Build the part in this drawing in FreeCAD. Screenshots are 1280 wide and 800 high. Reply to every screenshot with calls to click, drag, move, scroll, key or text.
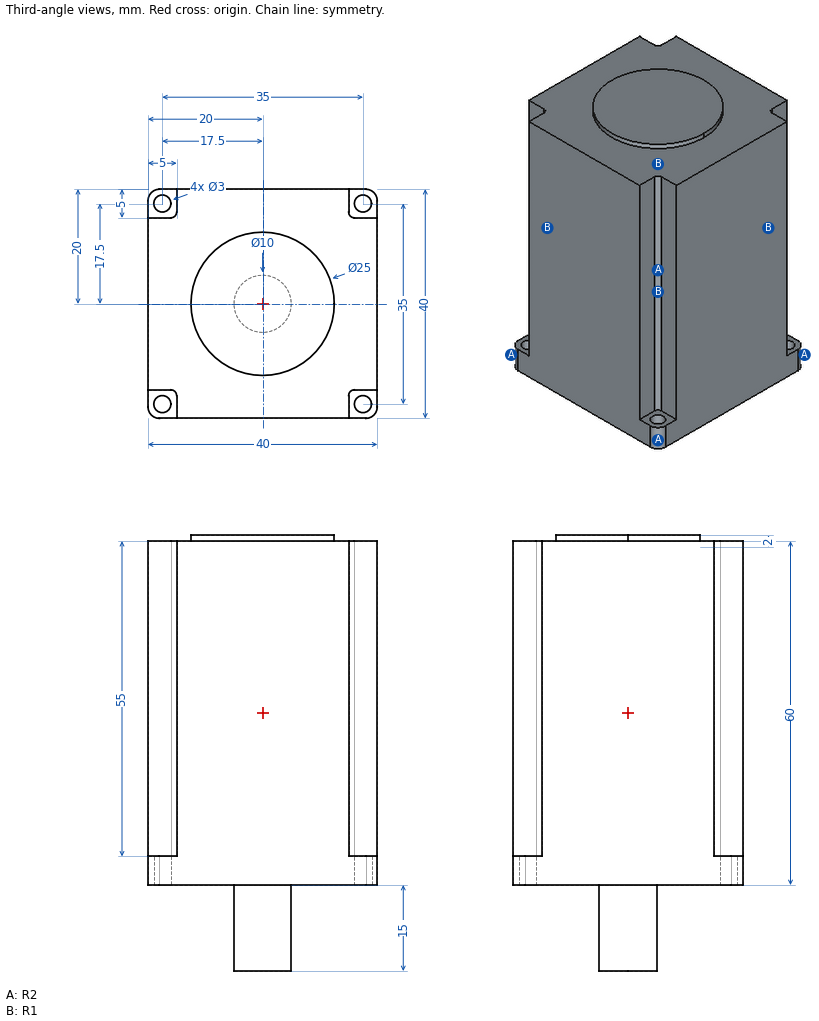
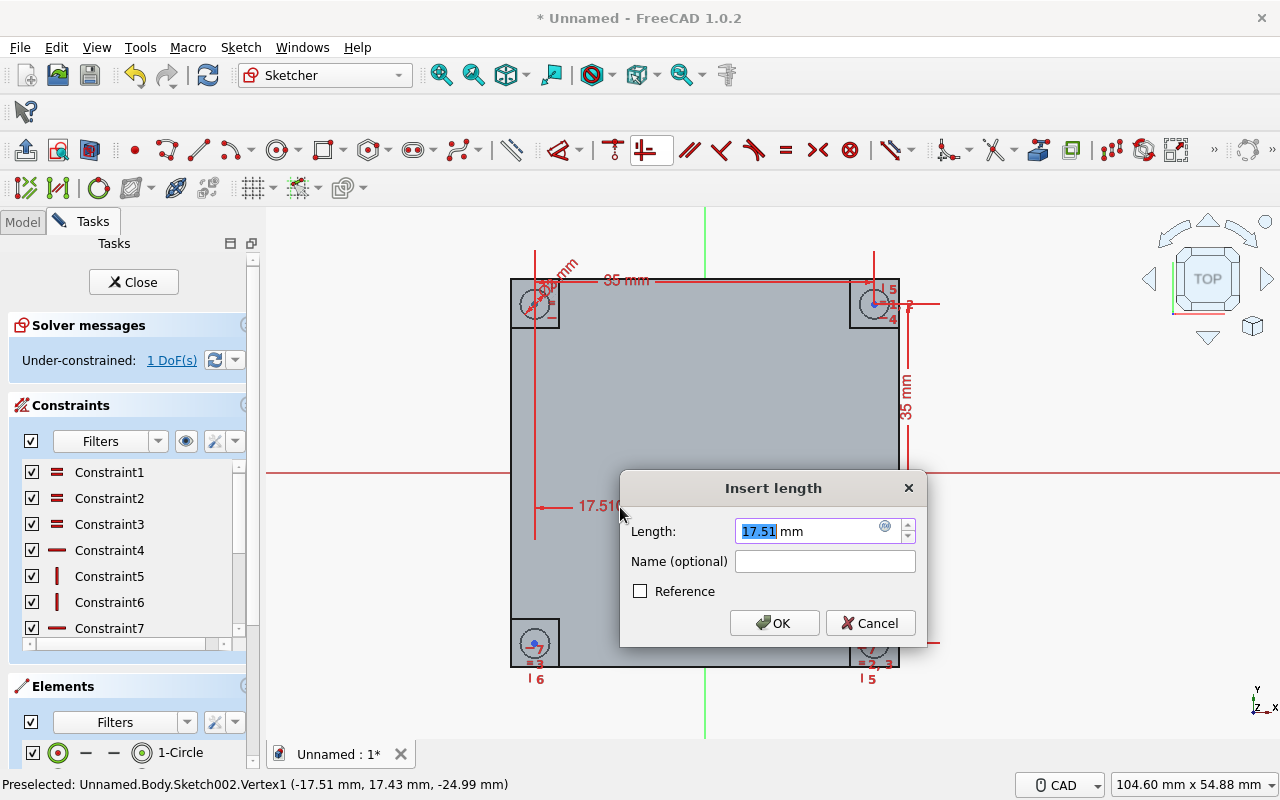
text(17.5)
key(Return)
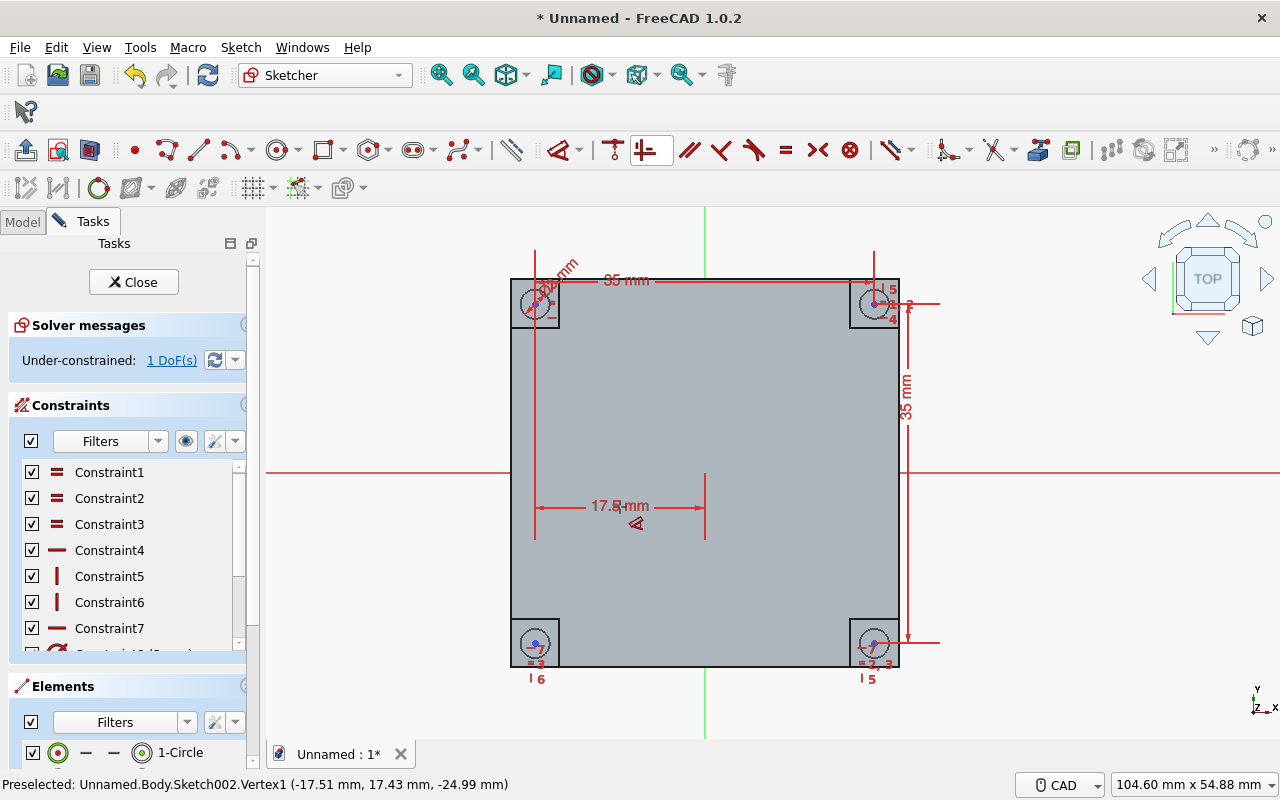
click(535, 304)
click(501, 389)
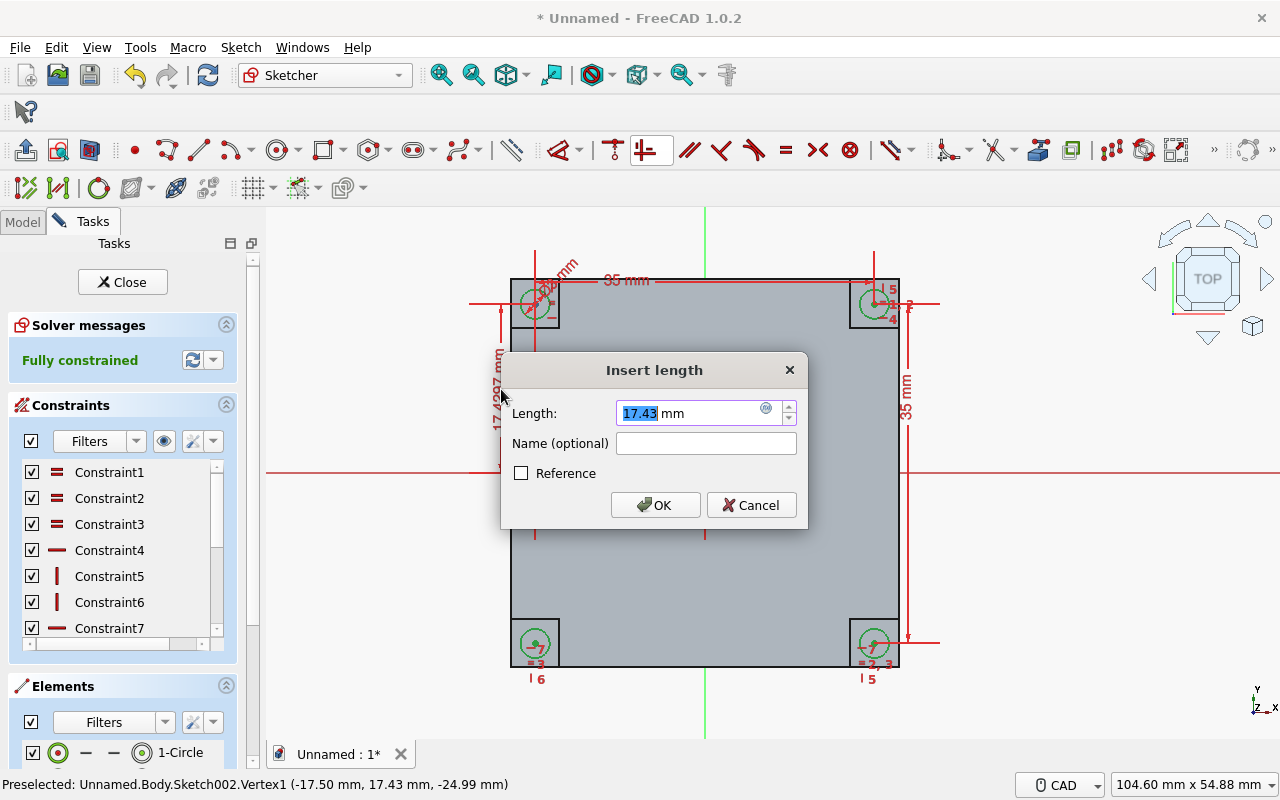
text(17.5)
key(Return)
key(Escape)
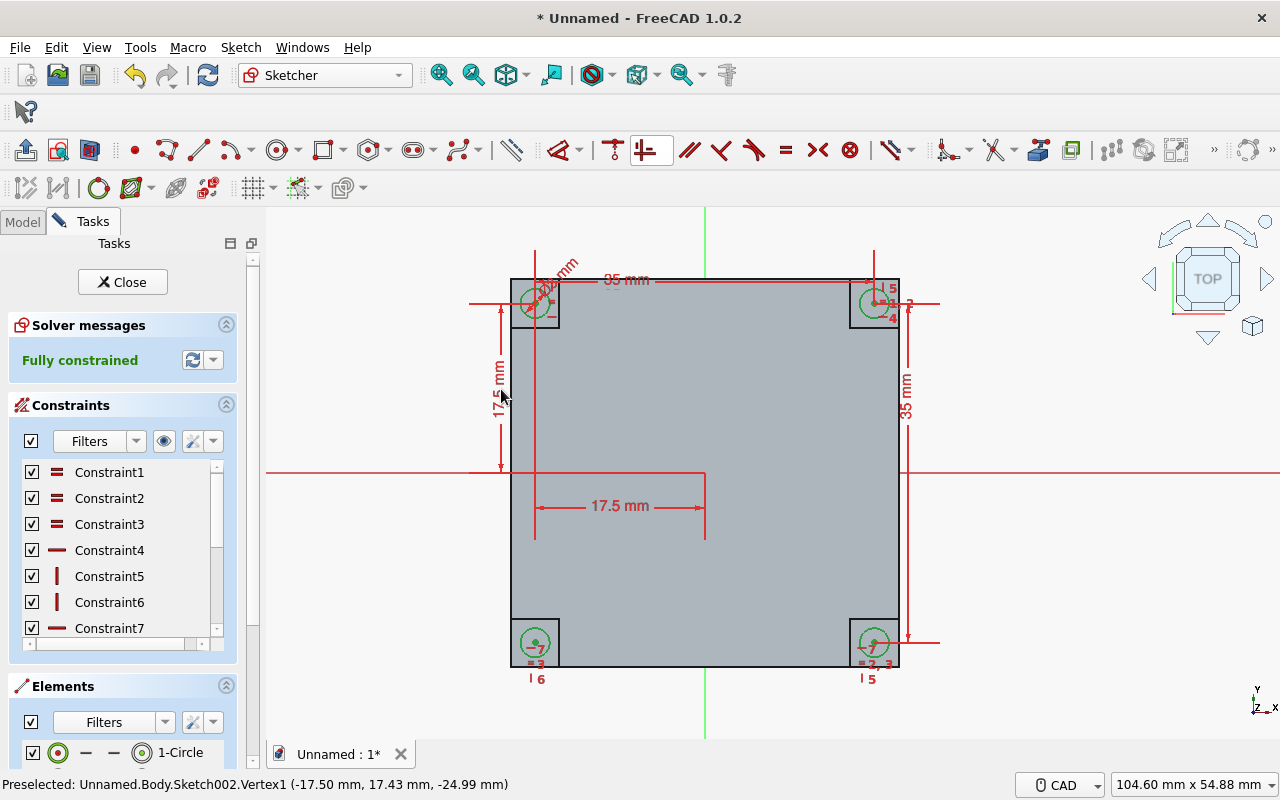
click(123, 282)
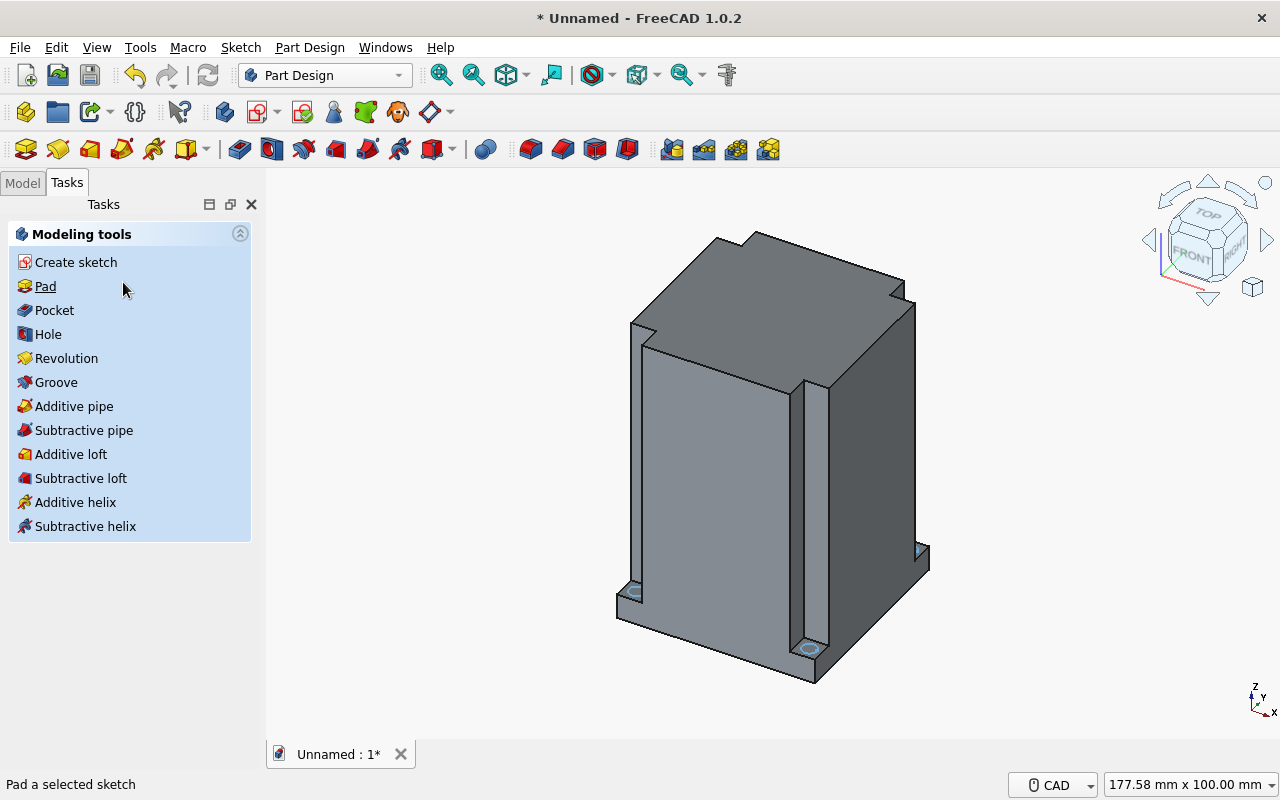
click(240, 150)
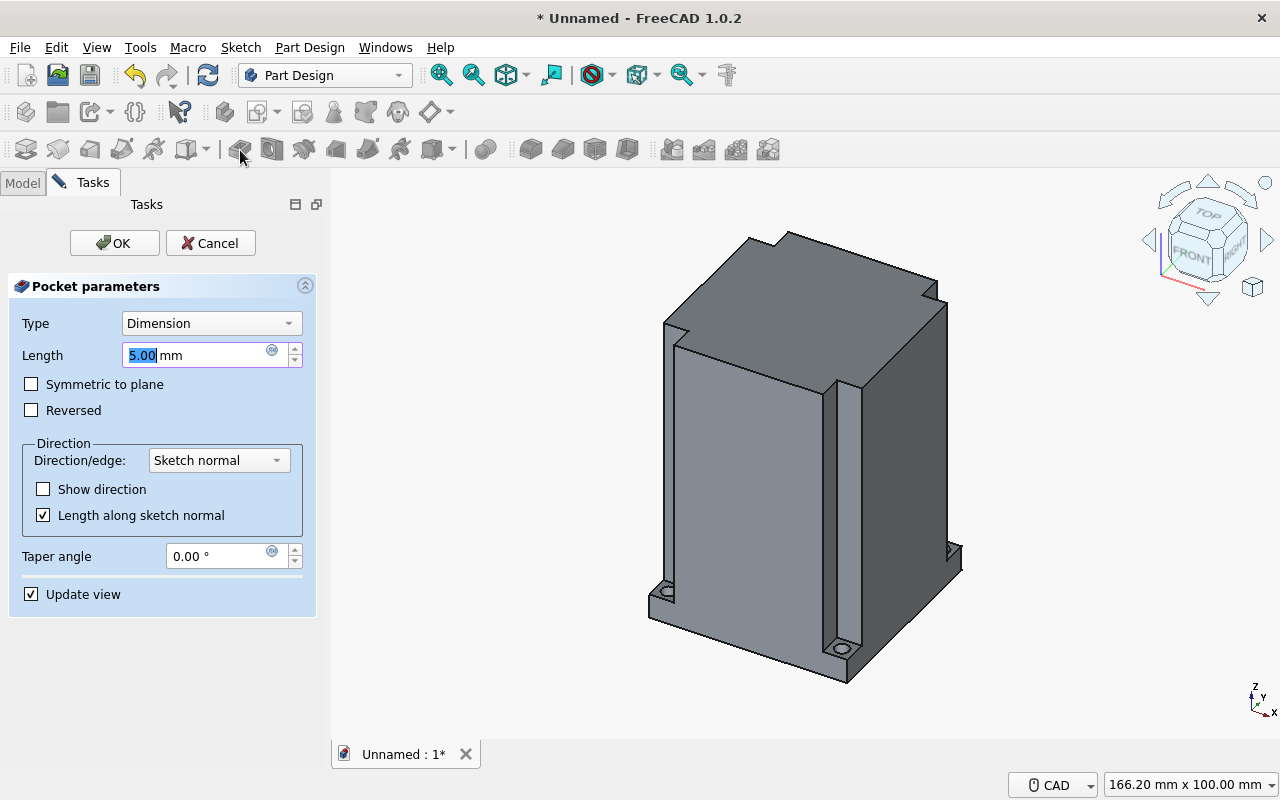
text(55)
key(Tab)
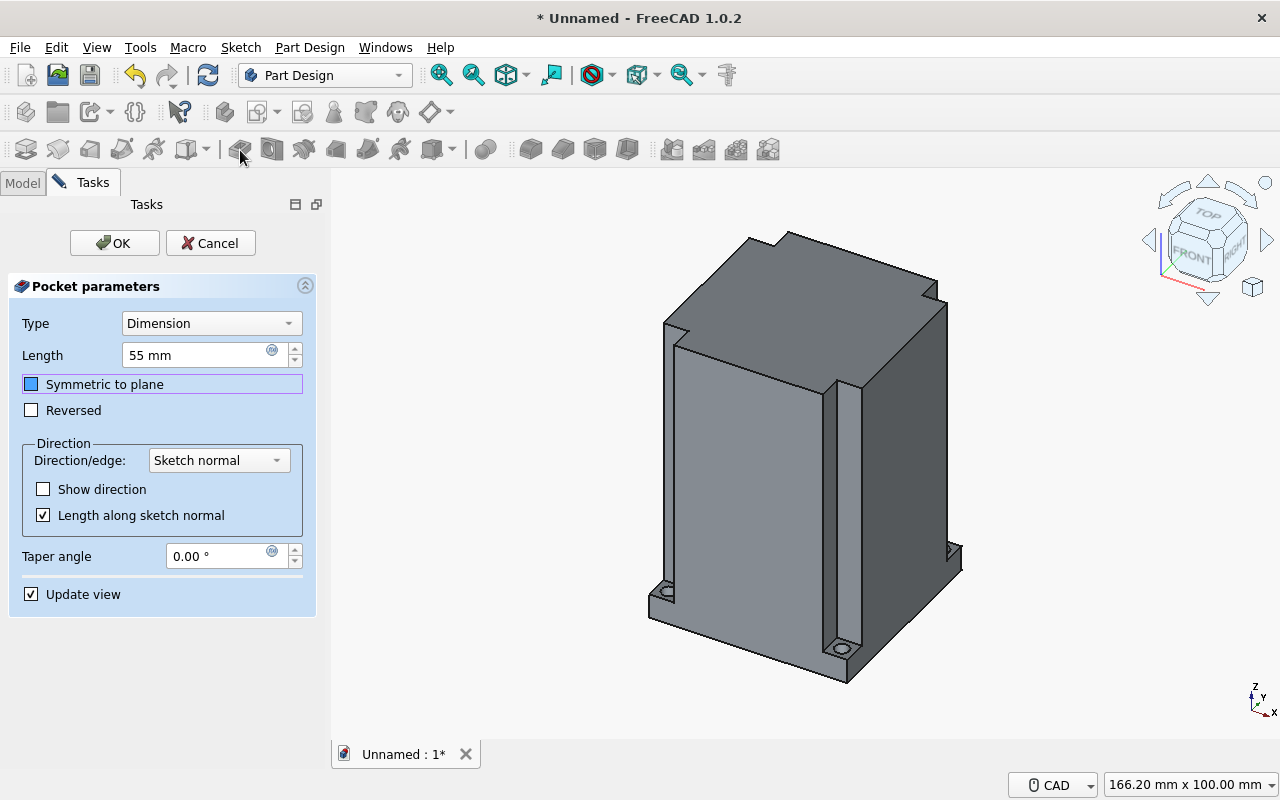
click(115, 243)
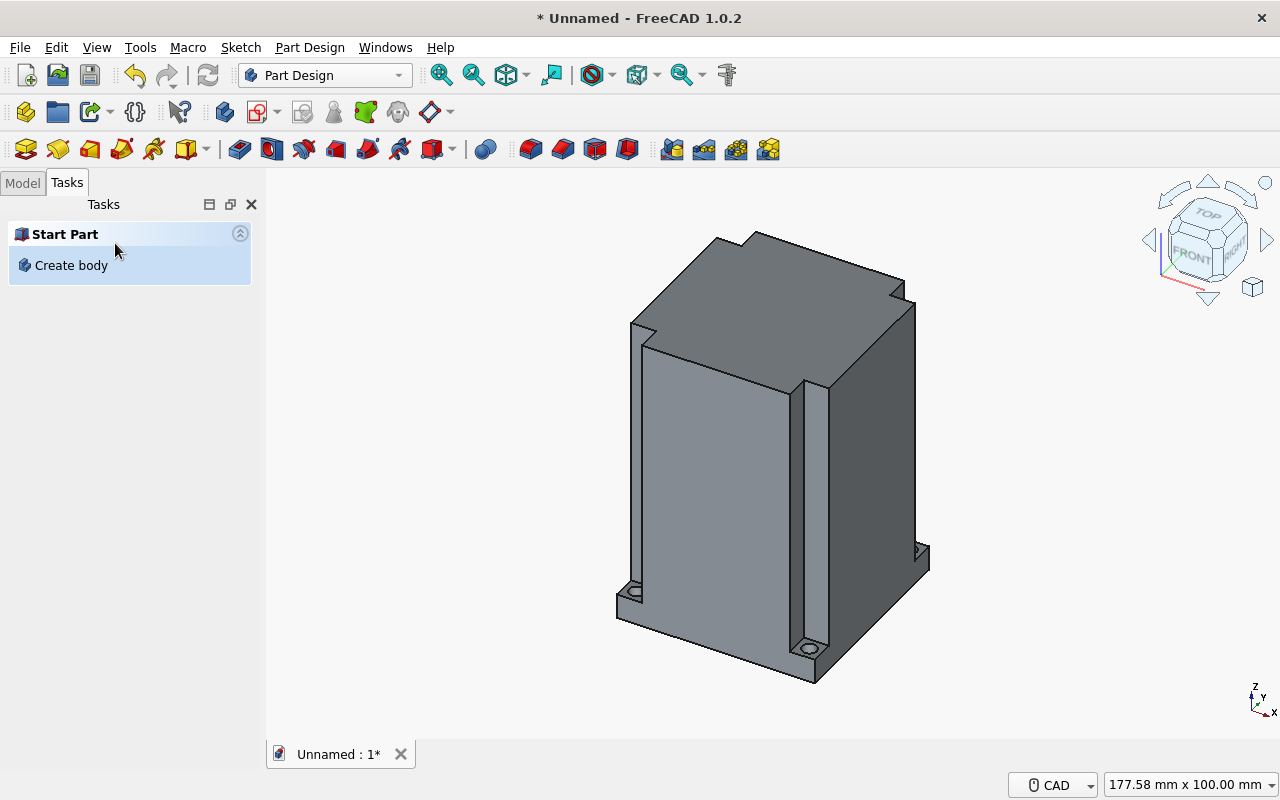
click(815, 671)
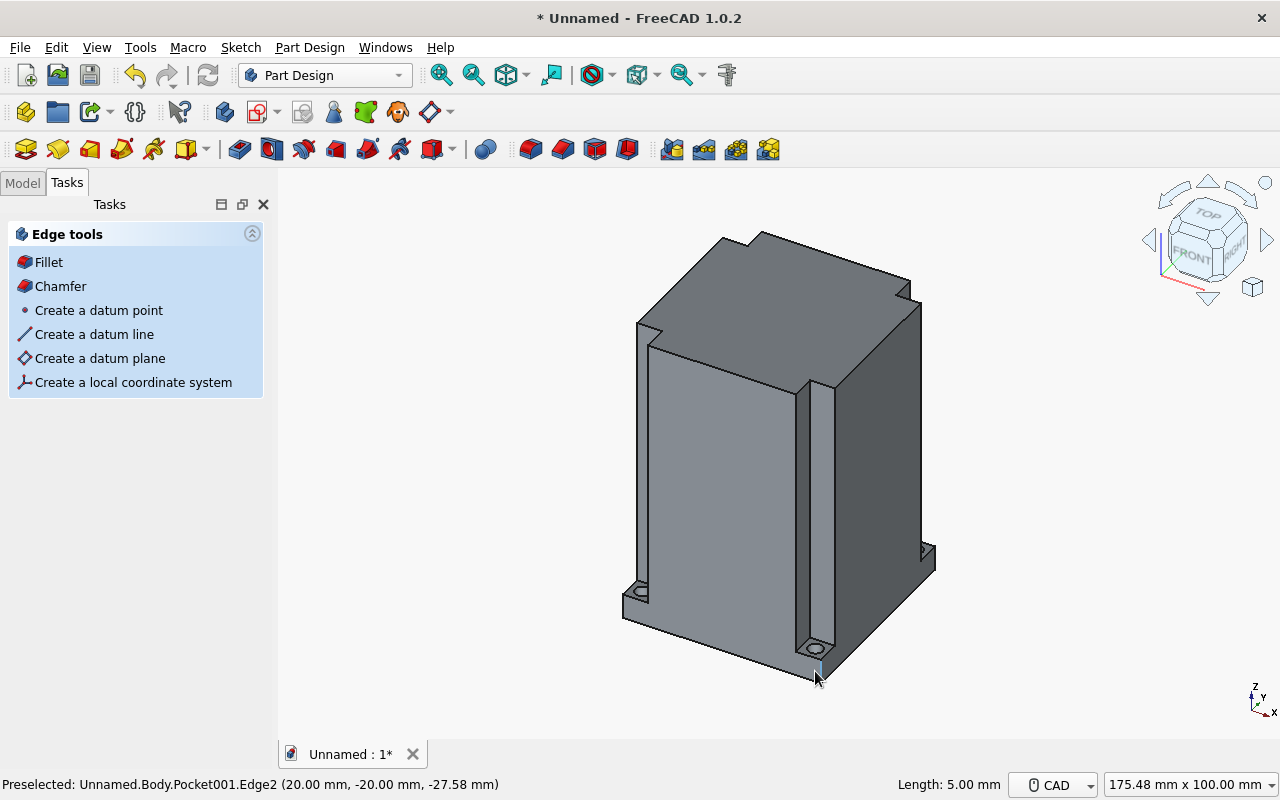
key(0)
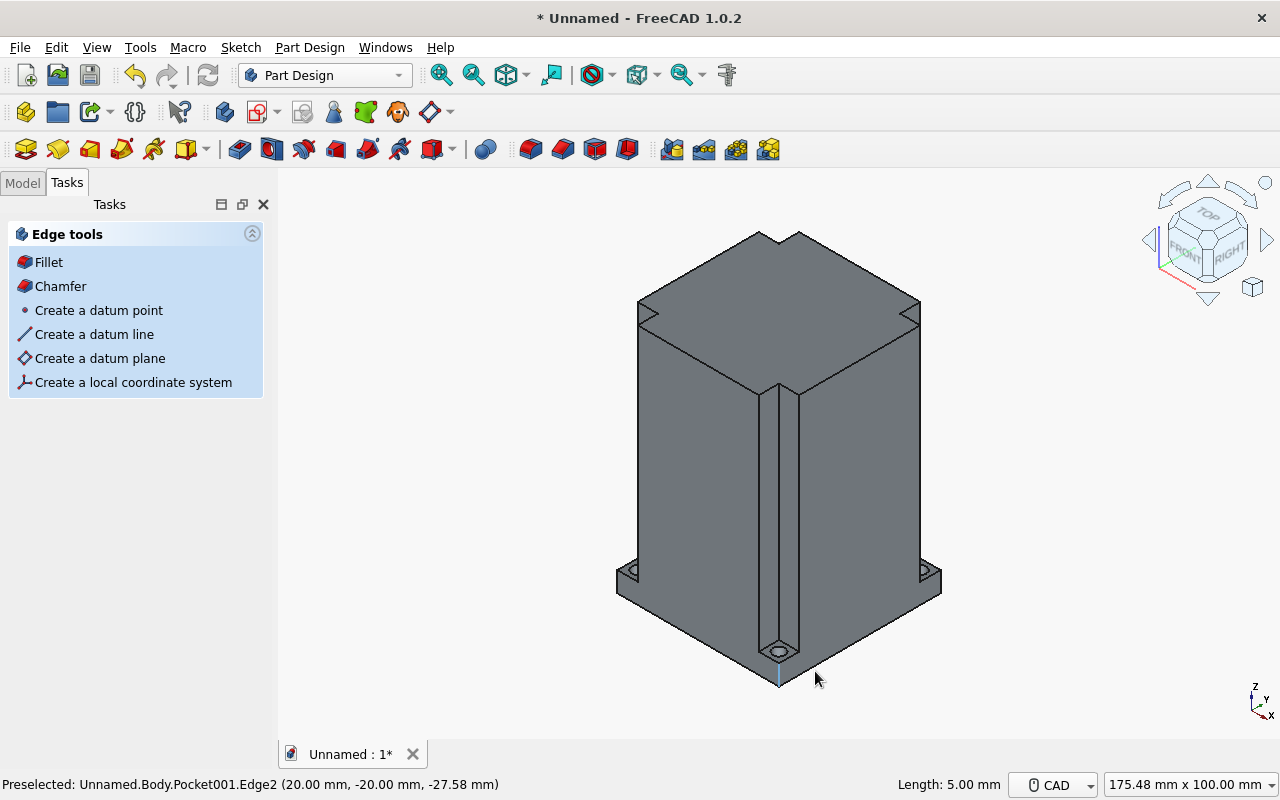
key(2)